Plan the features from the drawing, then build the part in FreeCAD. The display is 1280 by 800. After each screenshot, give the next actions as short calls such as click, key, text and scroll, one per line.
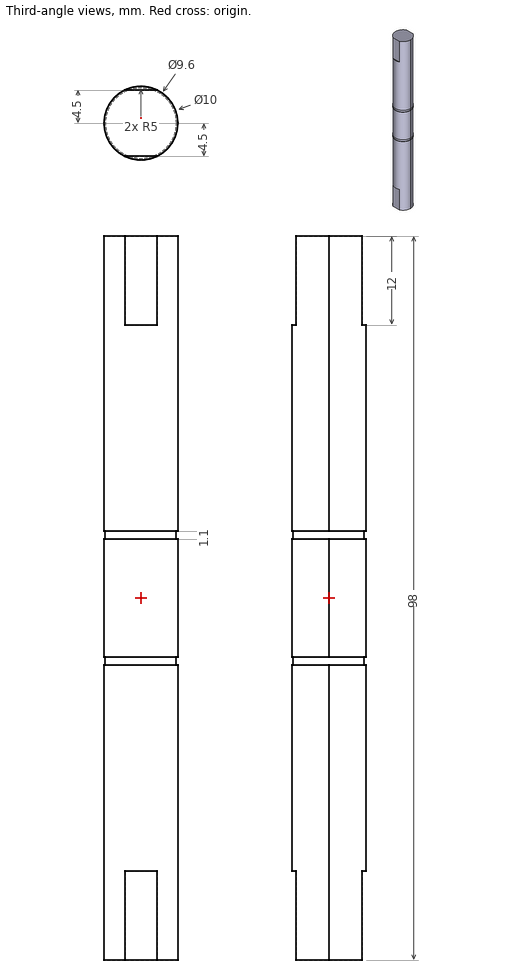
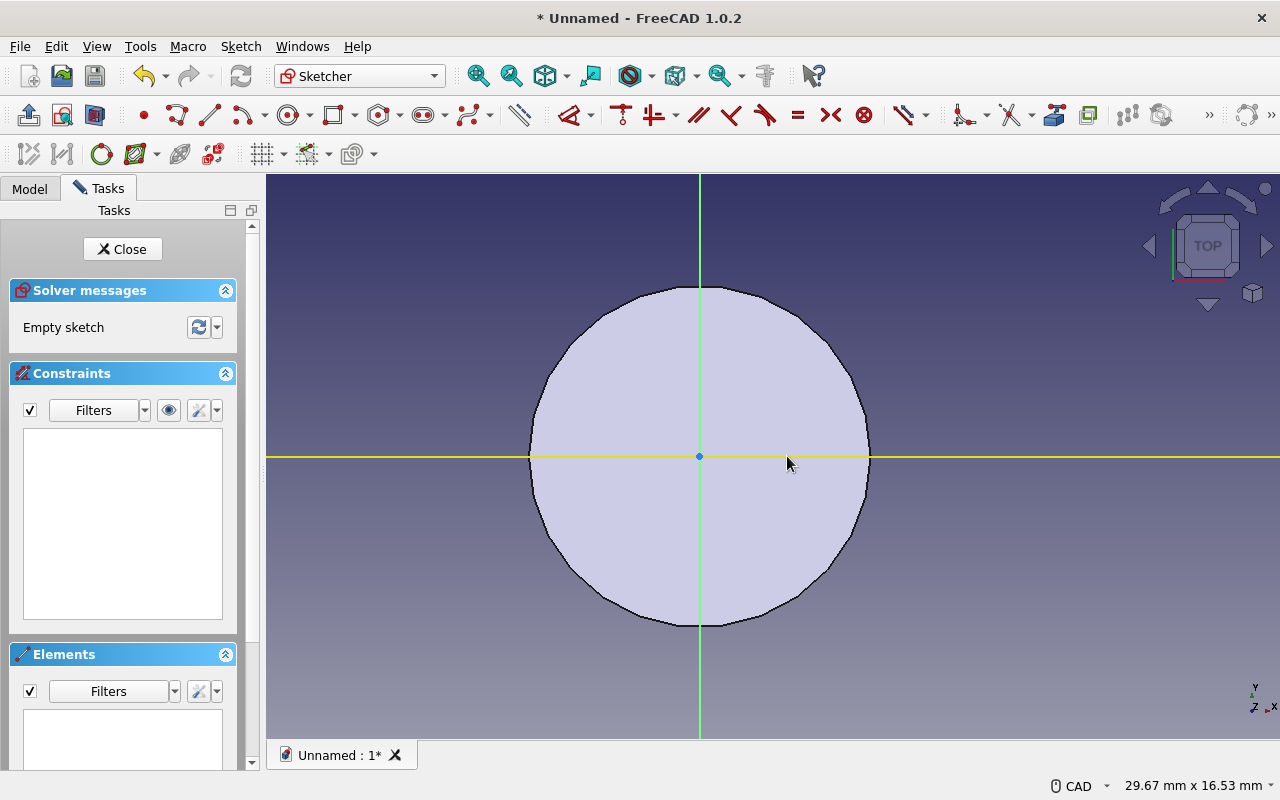
click(210, 116)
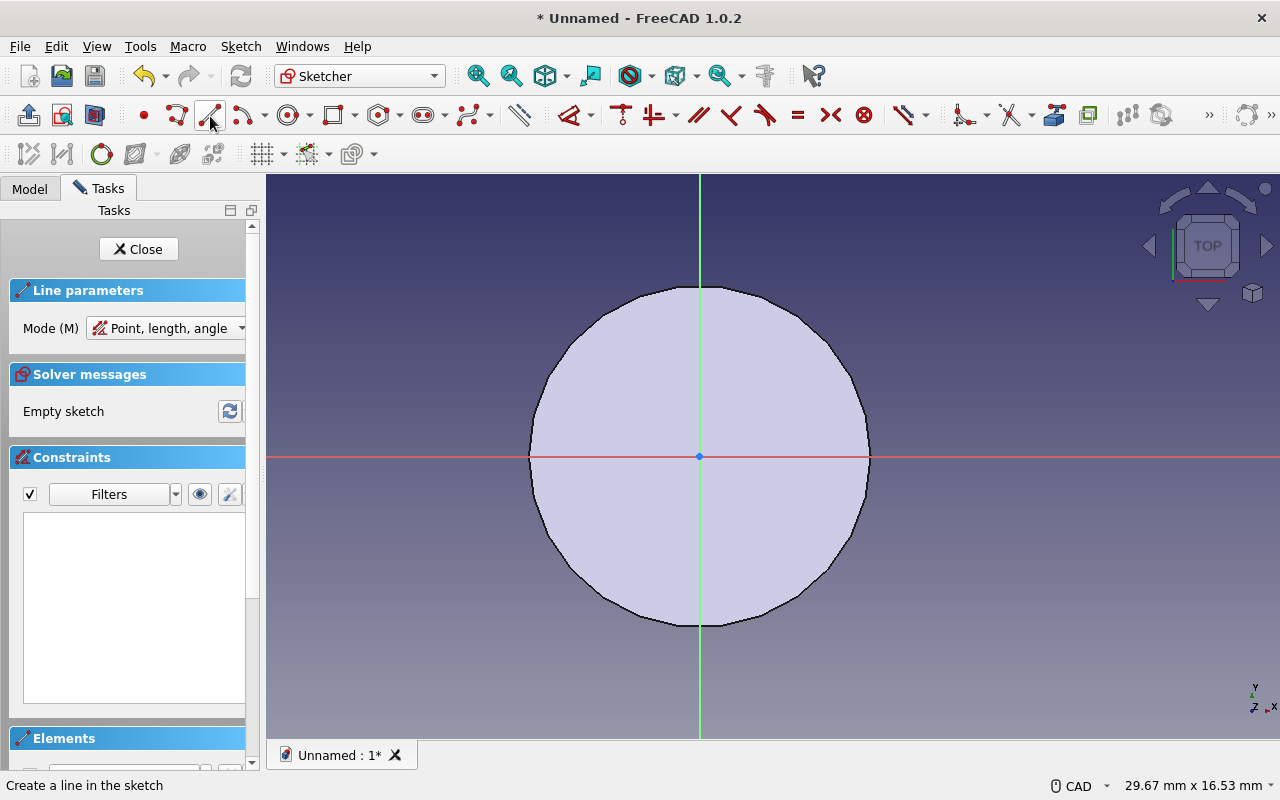
click(625, 303)
click(774, 303)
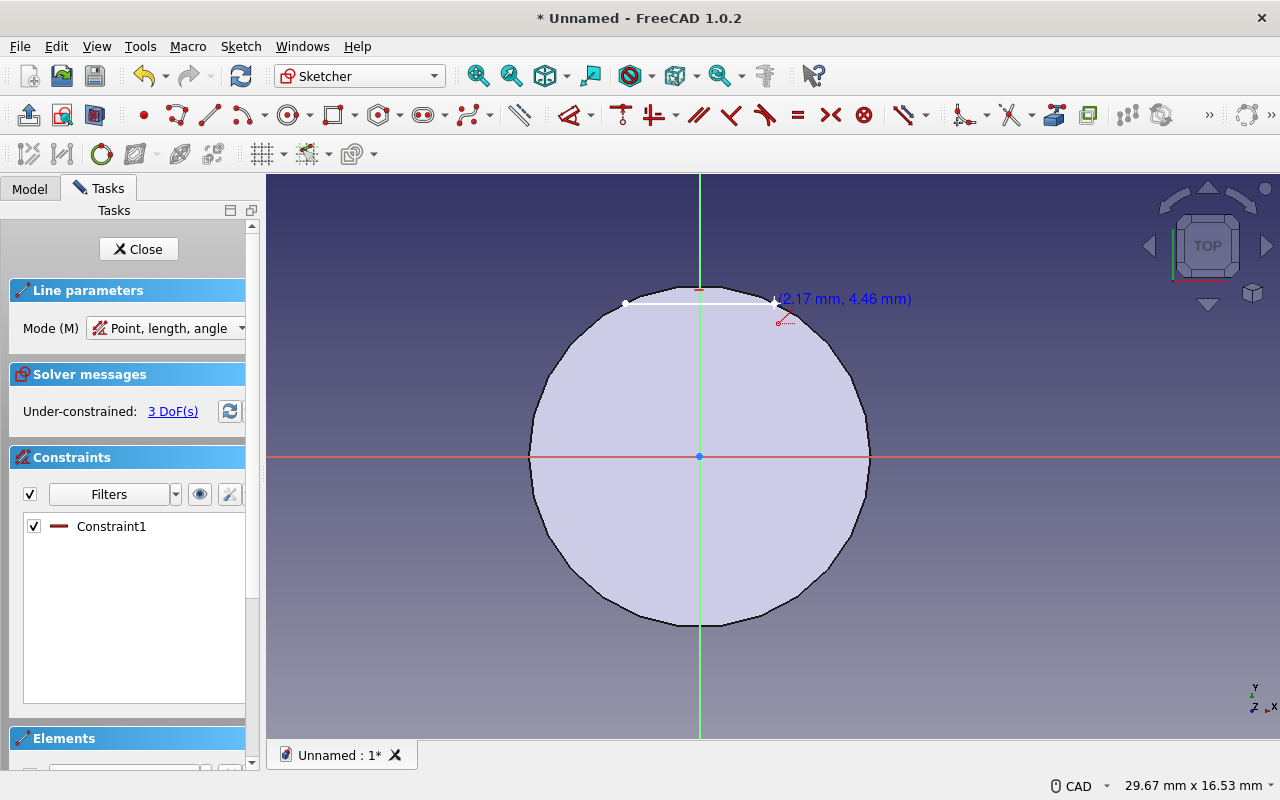
click(264, 116)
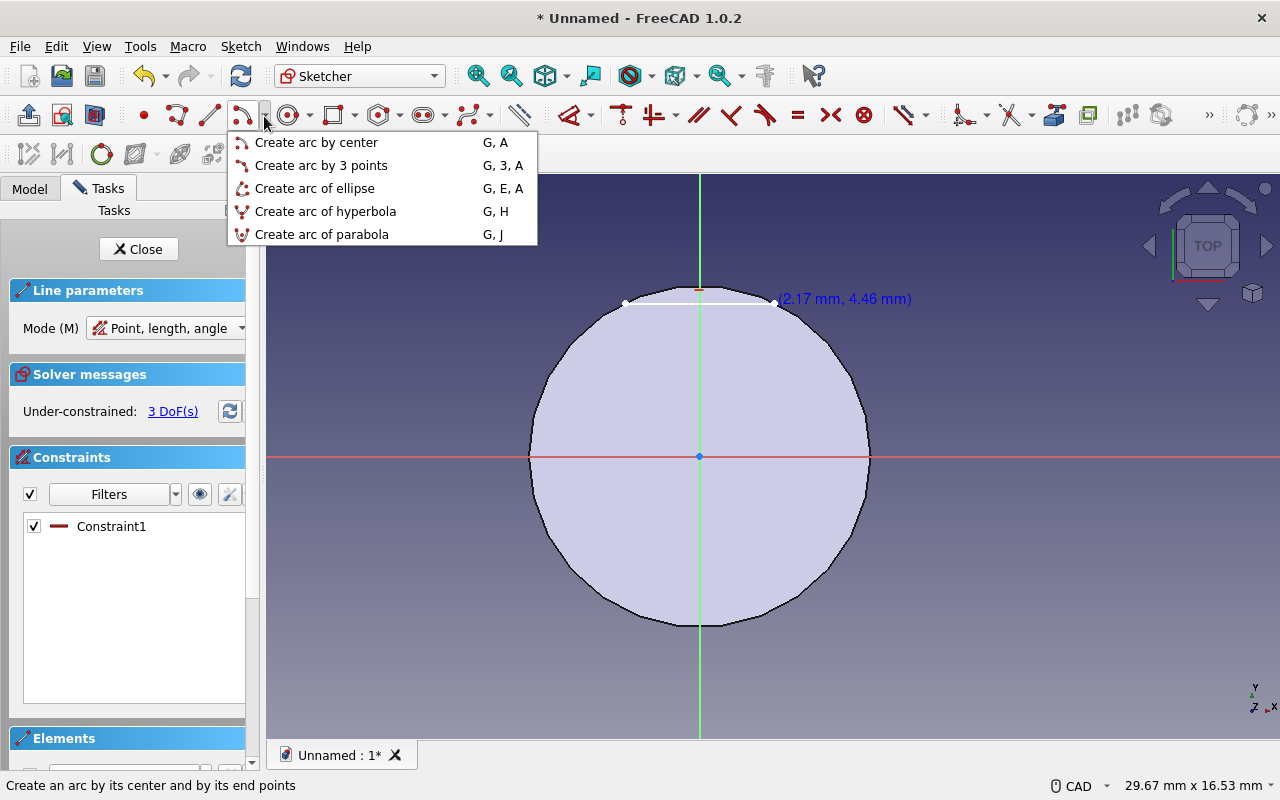
click(382, 166)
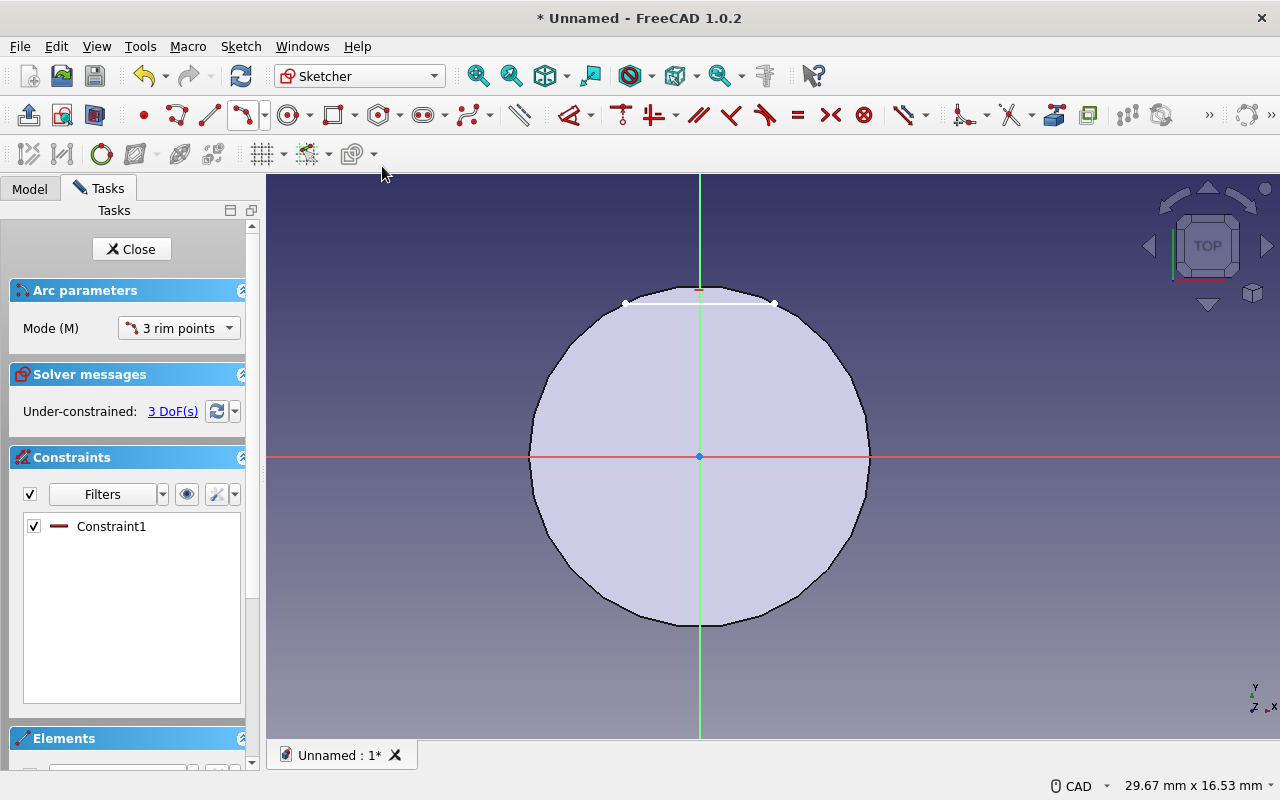
click(774, 304)
click(625, 304)
click(715, 286)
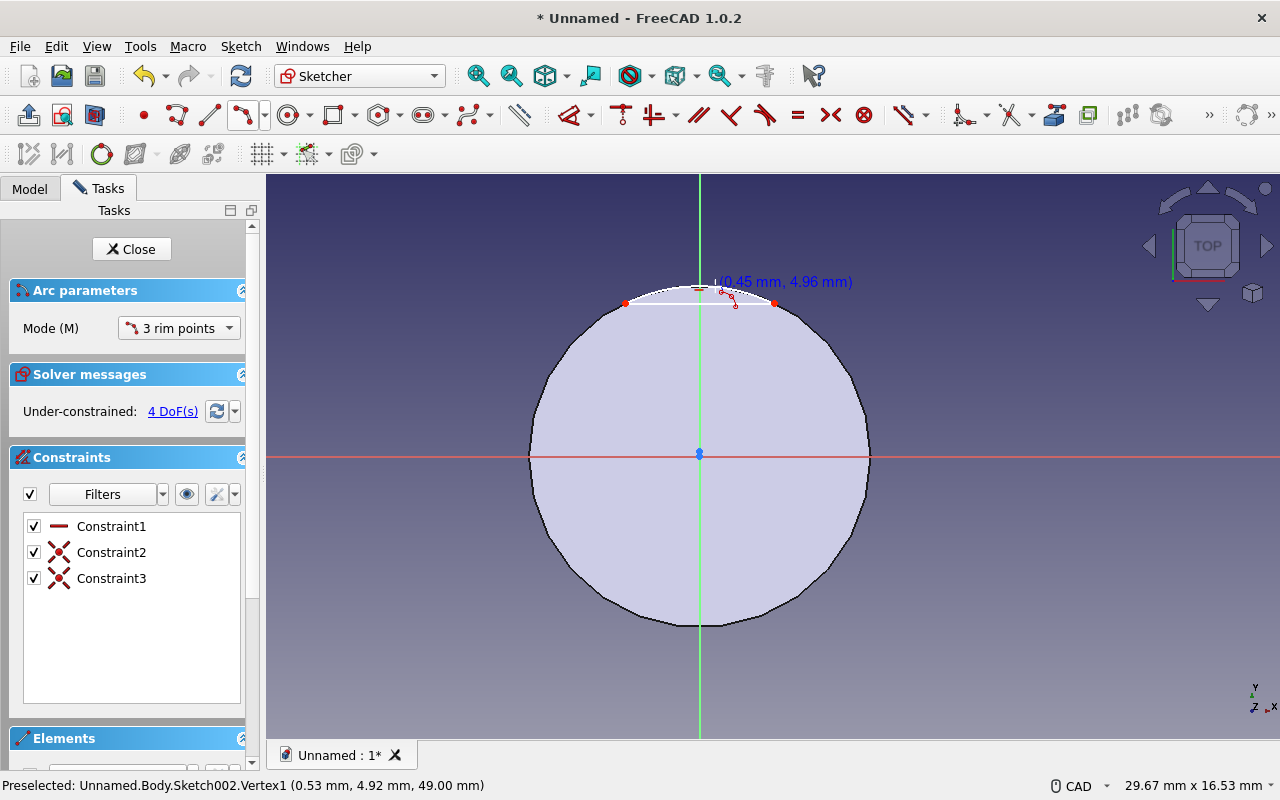
click(210, 116)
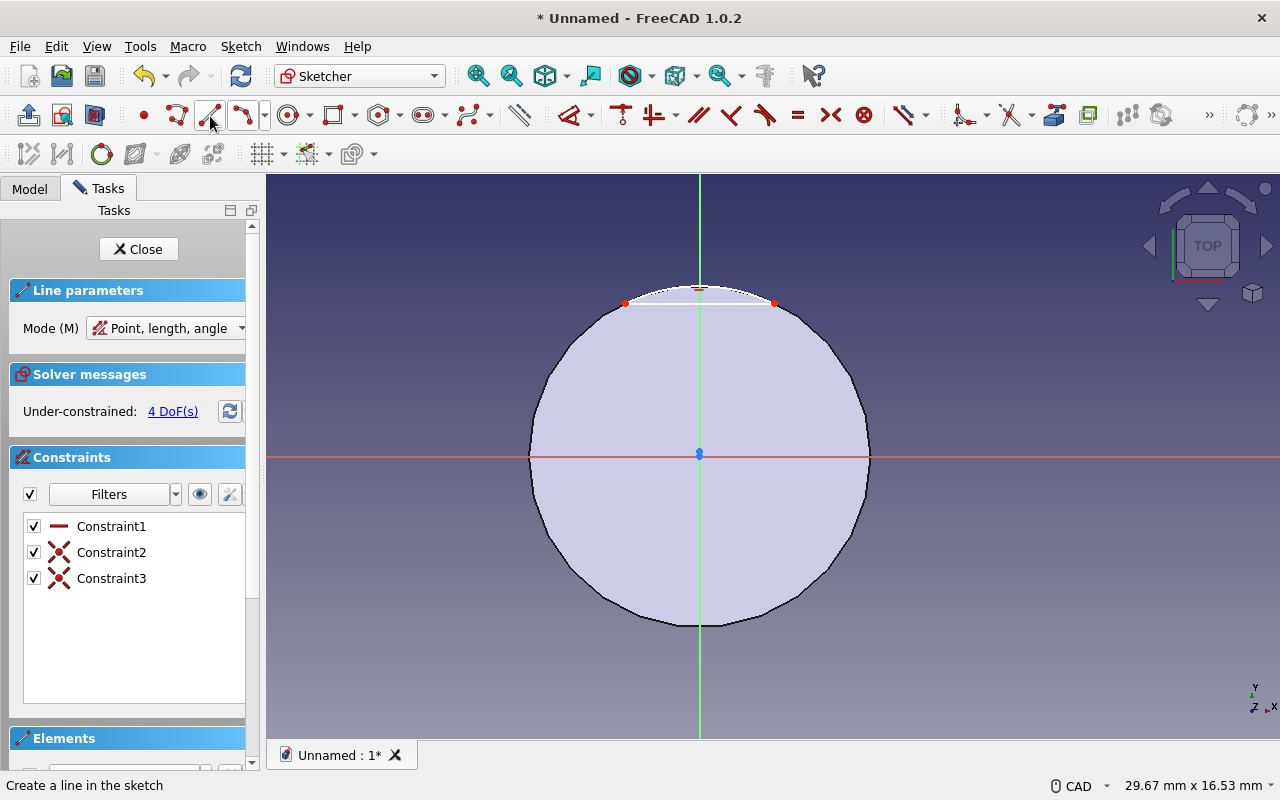
click(774, 610)
click(625, 610)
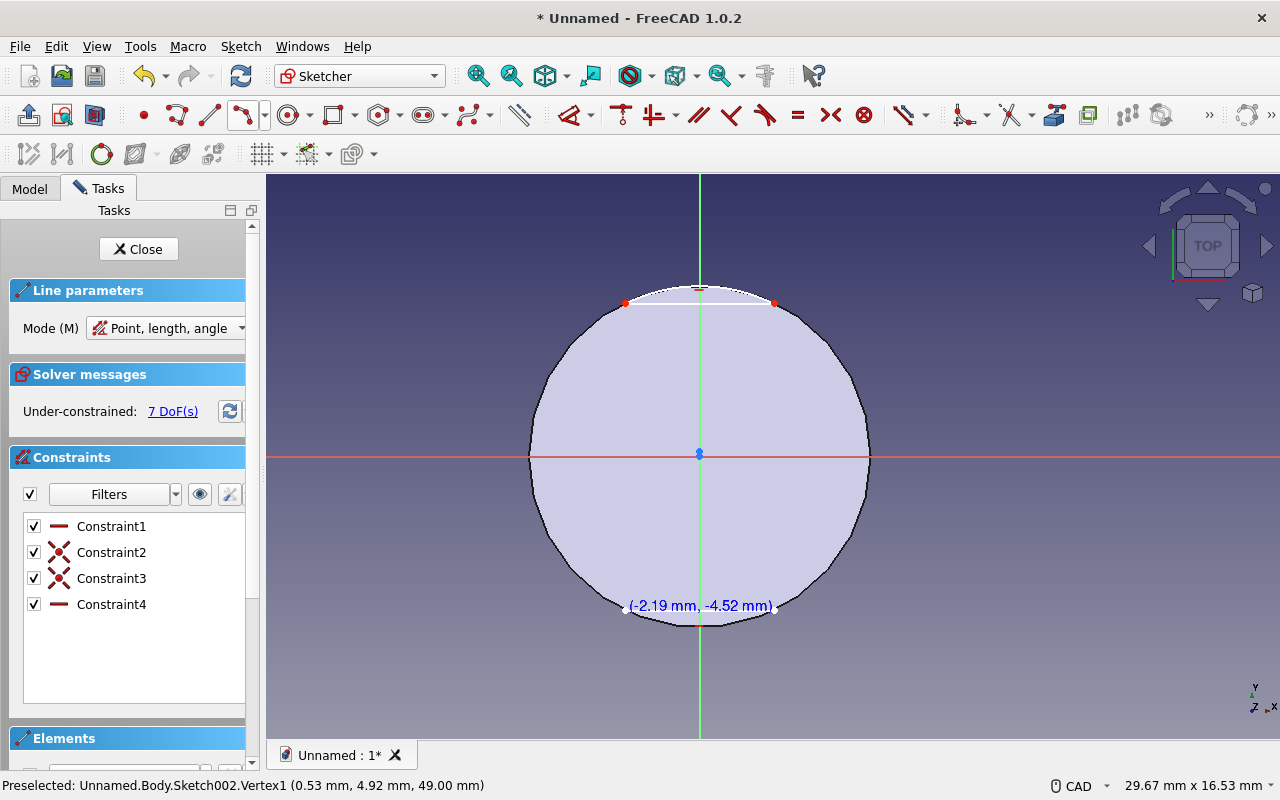
click(242, 116)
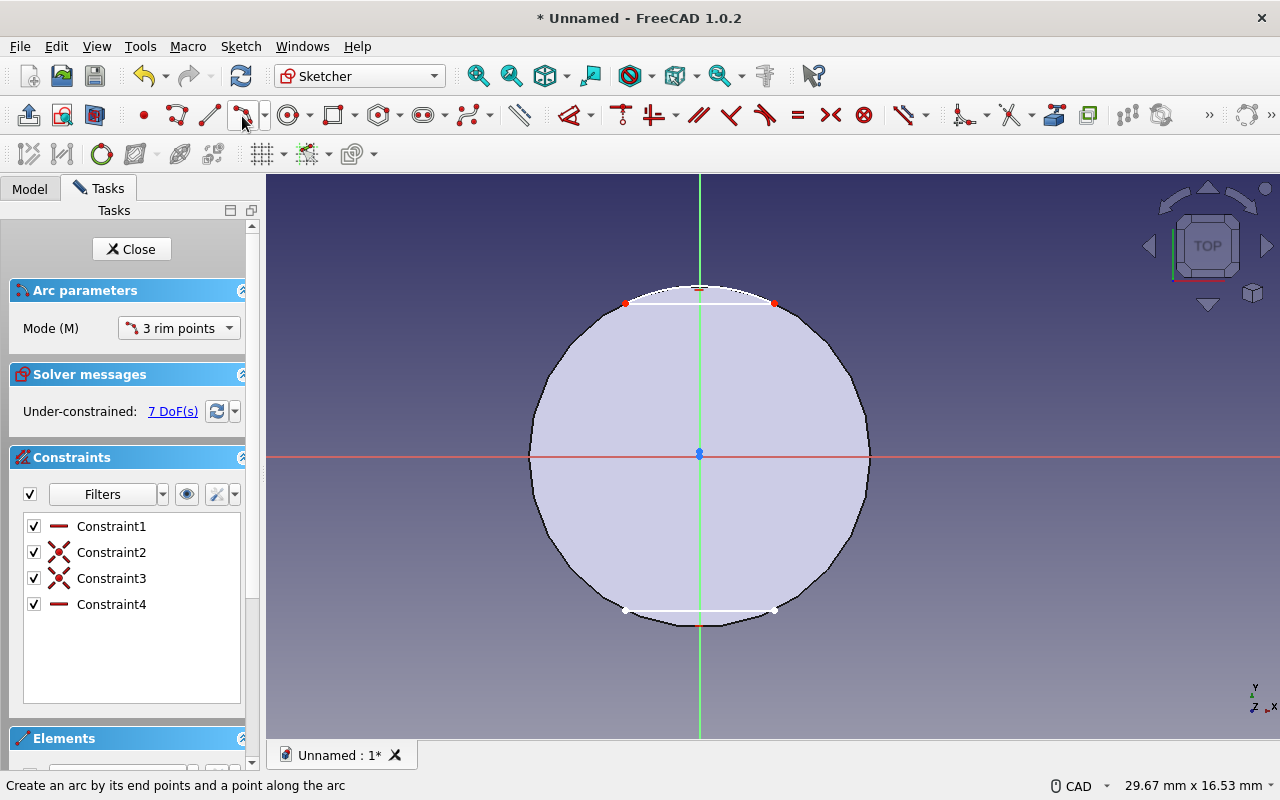
click(625, 611)
click(774, 611)
click(684, 627)
key(Escape)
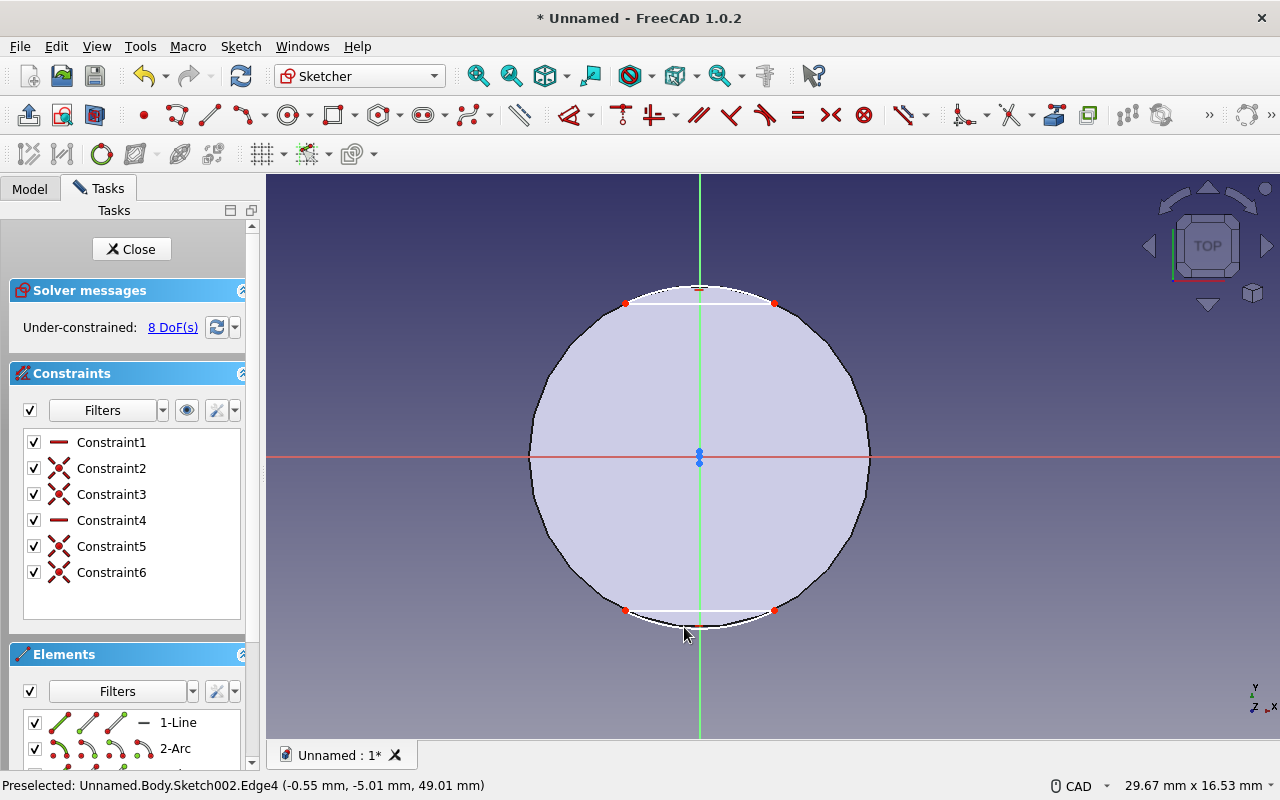
click(730, 289)